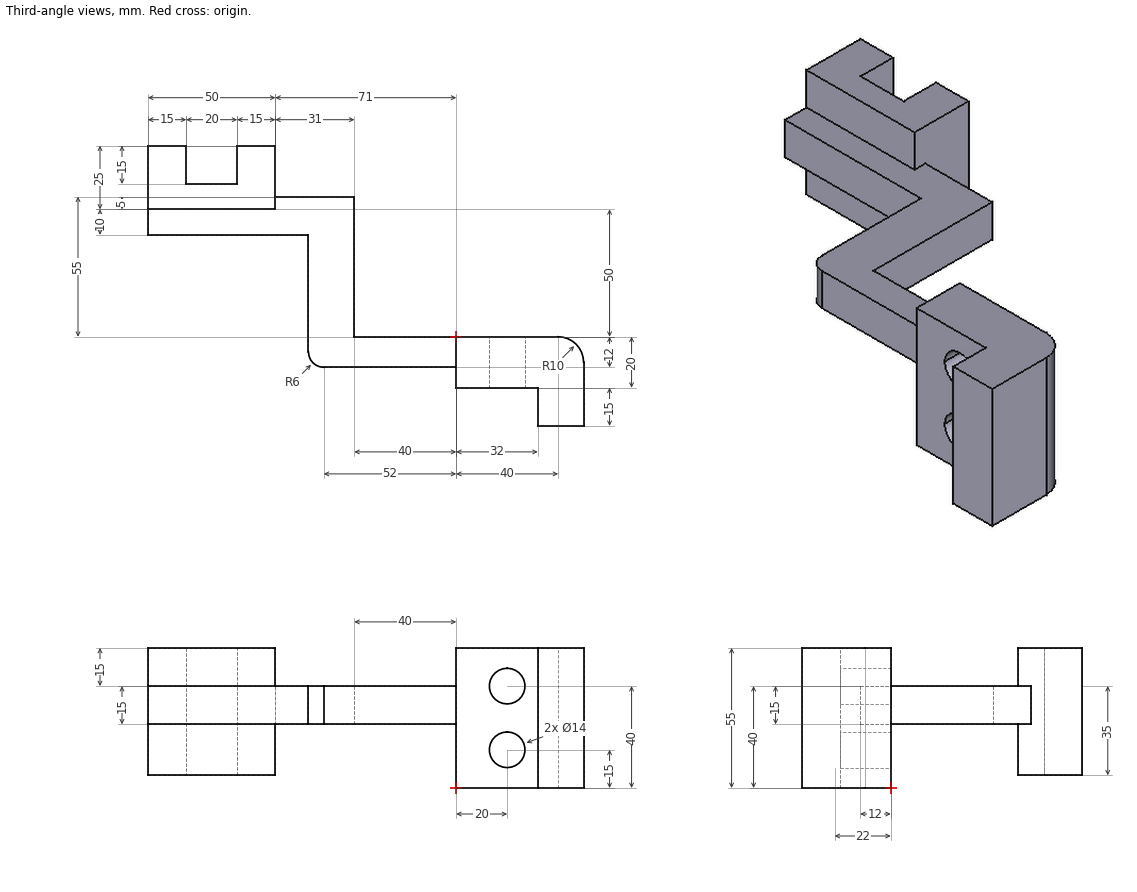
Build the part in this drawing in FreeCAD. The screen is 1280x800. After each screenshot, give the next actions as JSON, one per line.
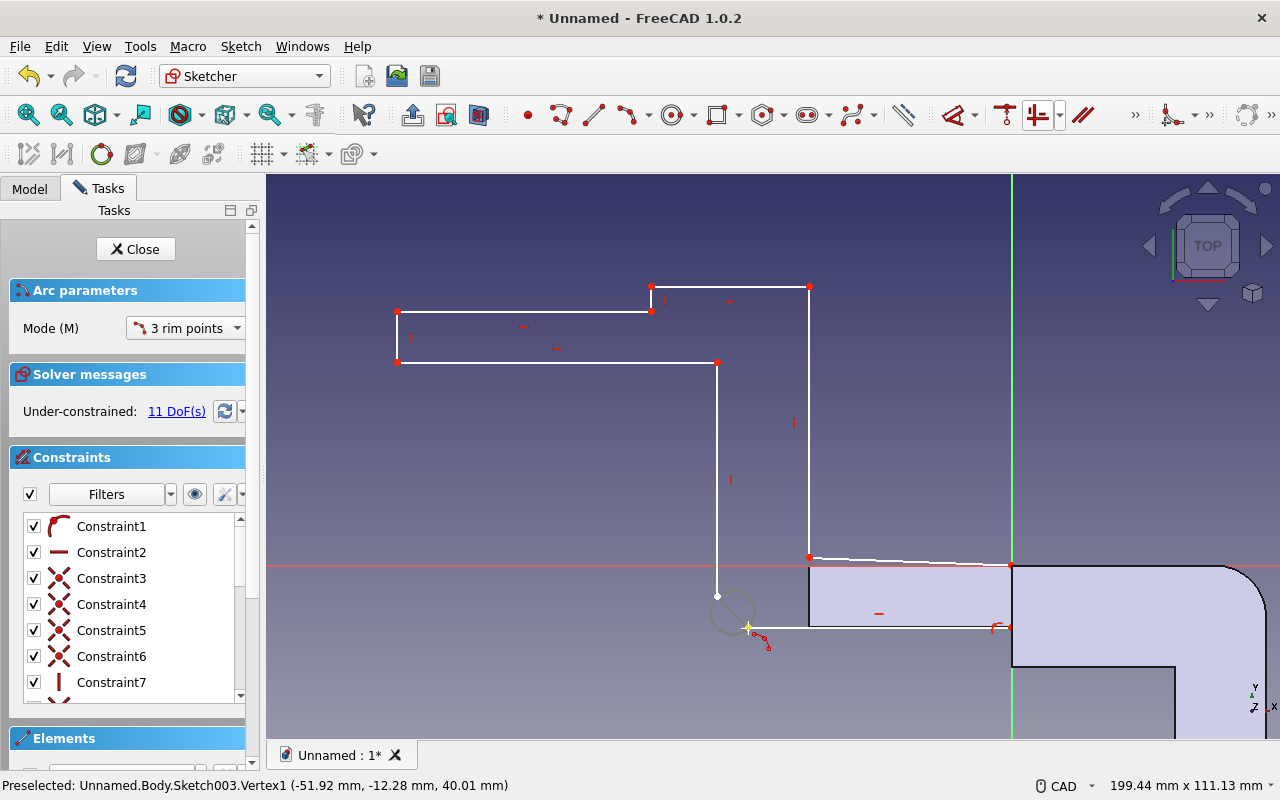
{"action": "scroll", "coordinate": [726, 618], "scroll_direction": "up", "scroll_amount": 3}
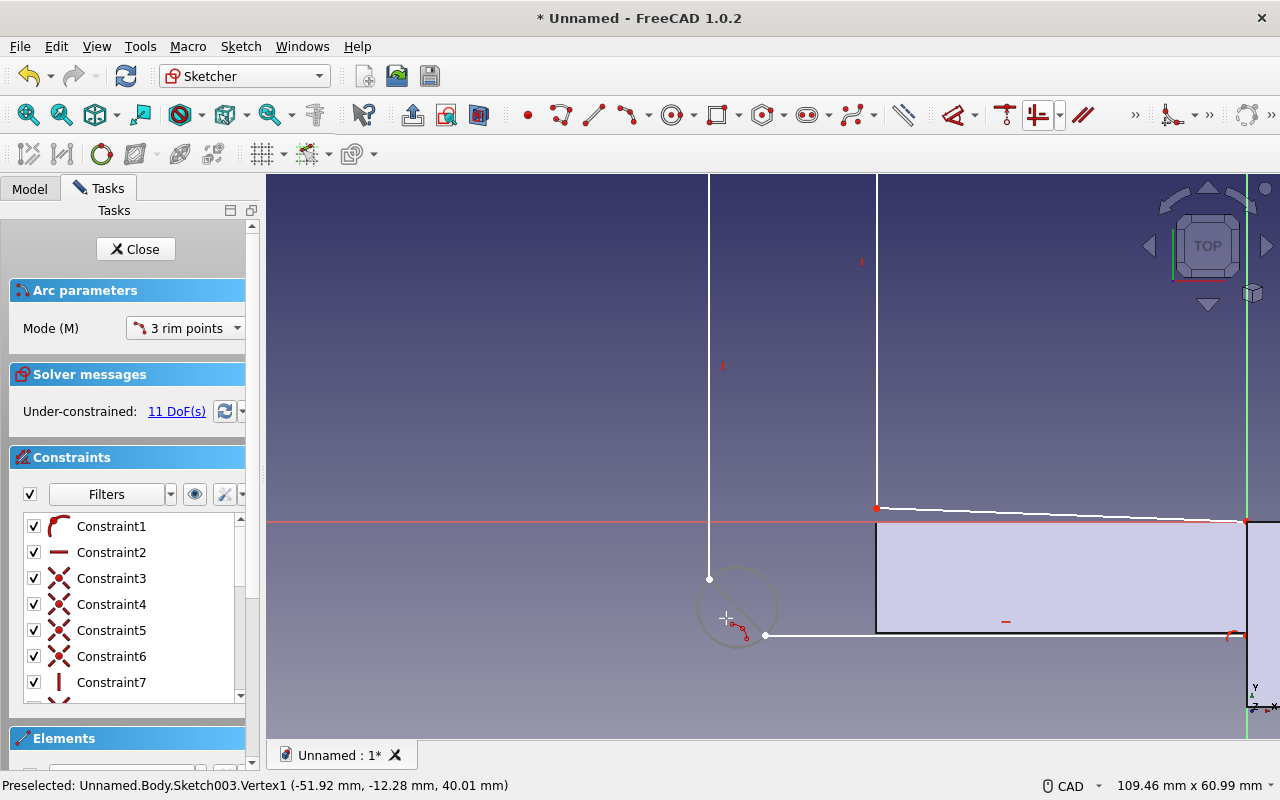
{"action": "left_click", "coordinate": [726, 617]}
{"action": "key", "text": "Escape"}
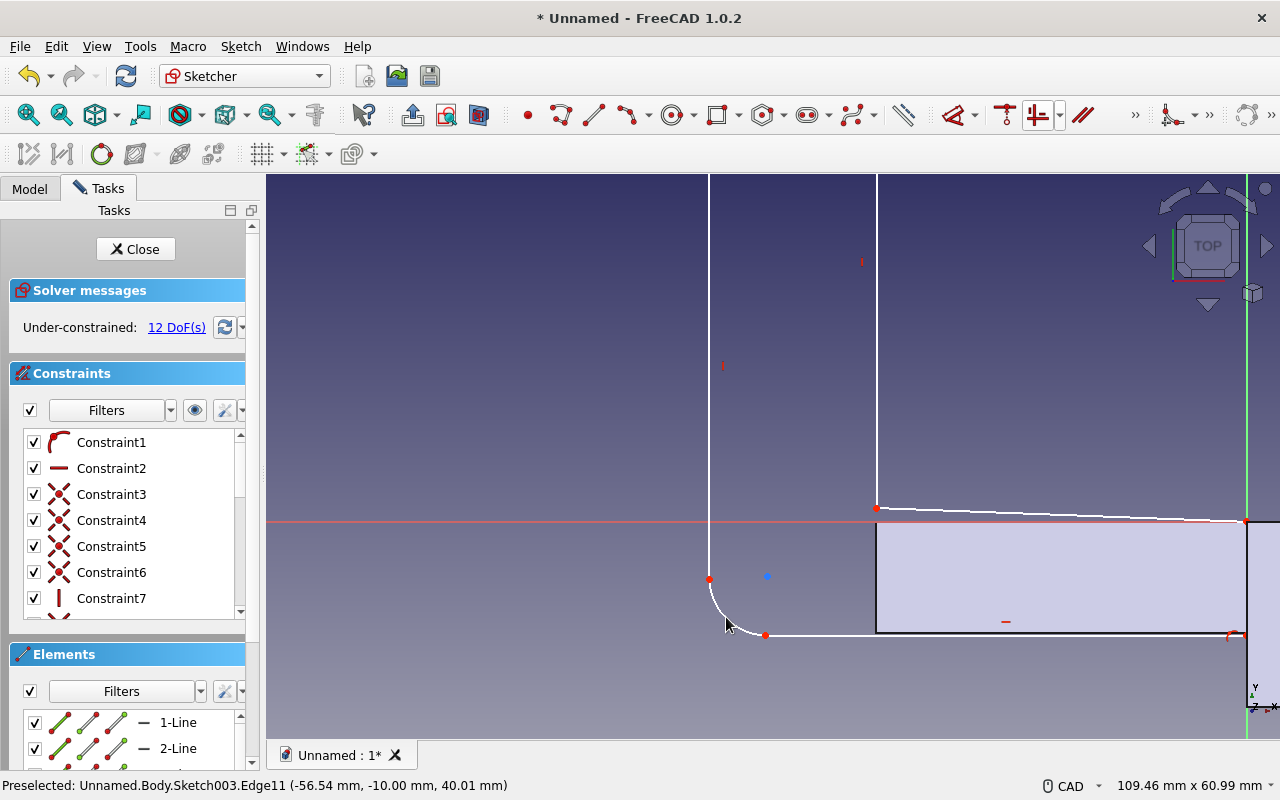
{"action": "left_click", "coordinate": [910, 636]}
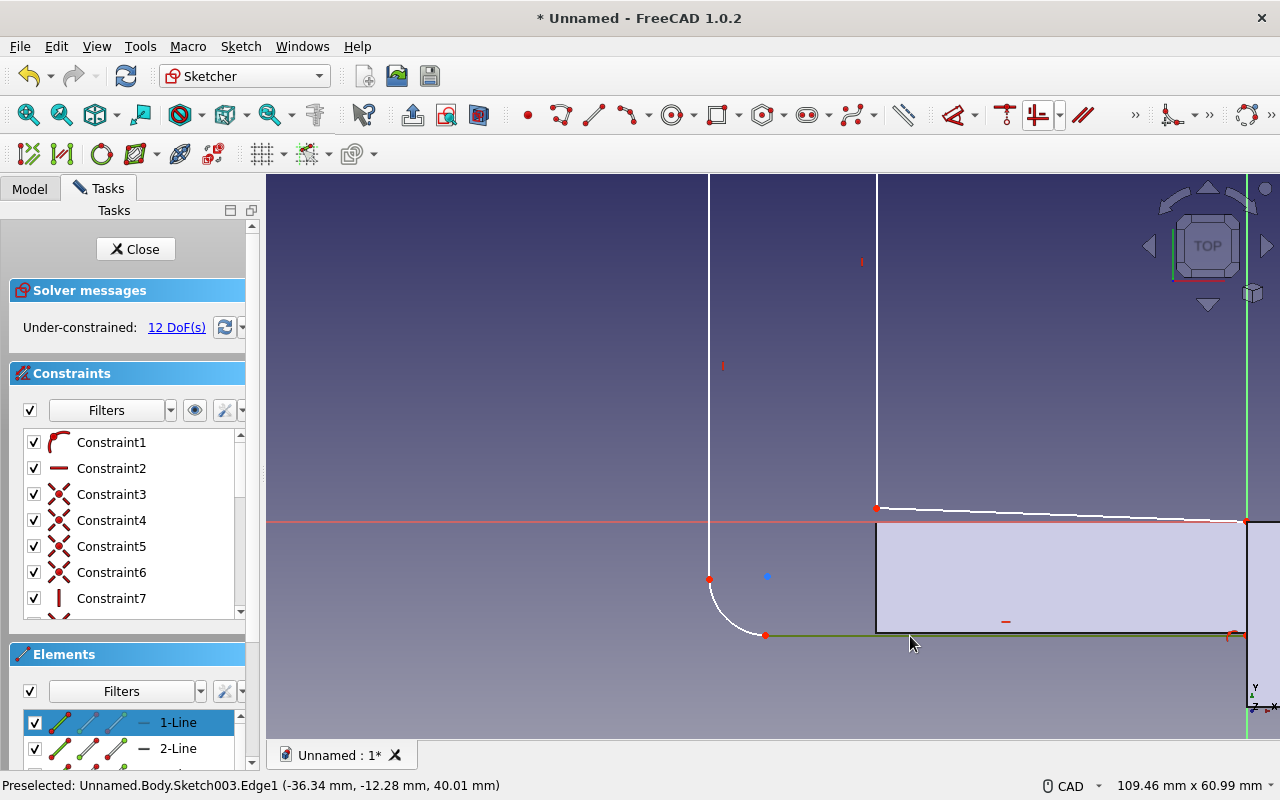
{"action": "left_click", "coordinate": [716, 604]}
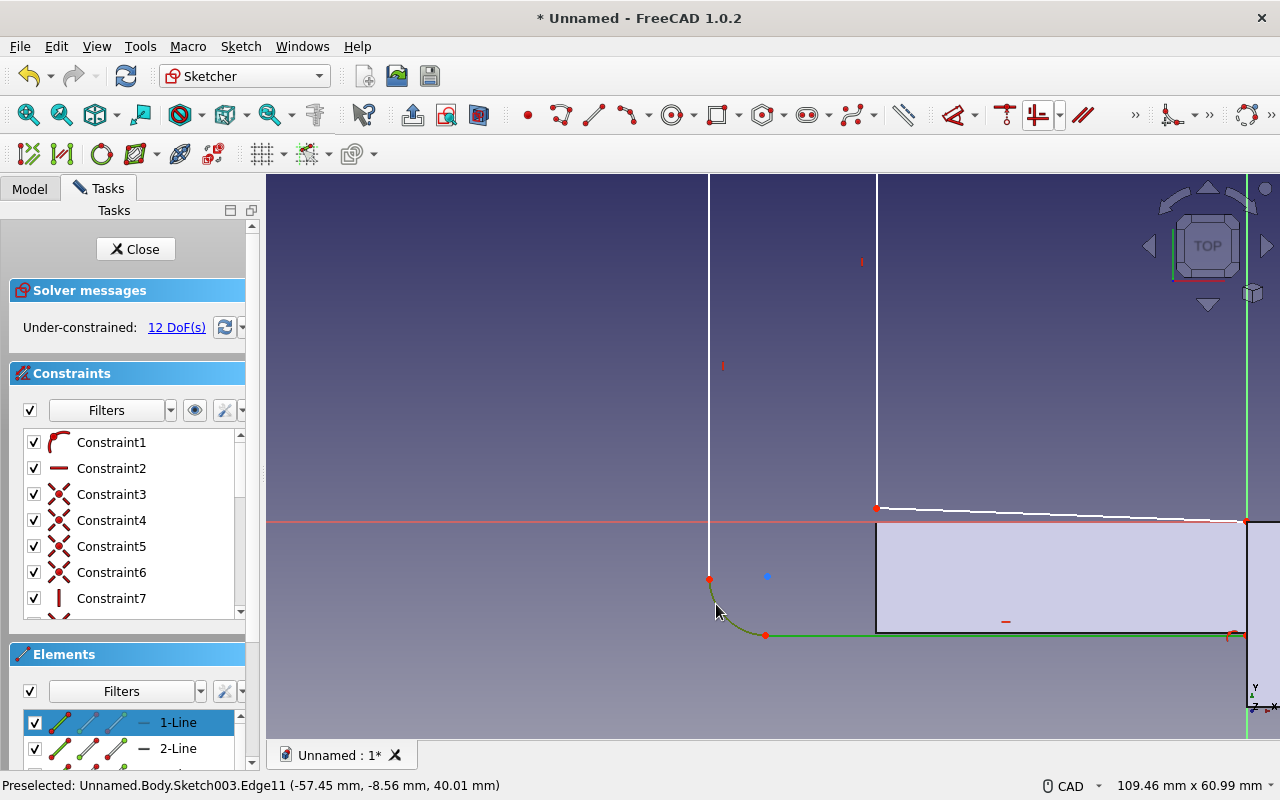
{"action": "key", "text": "t"}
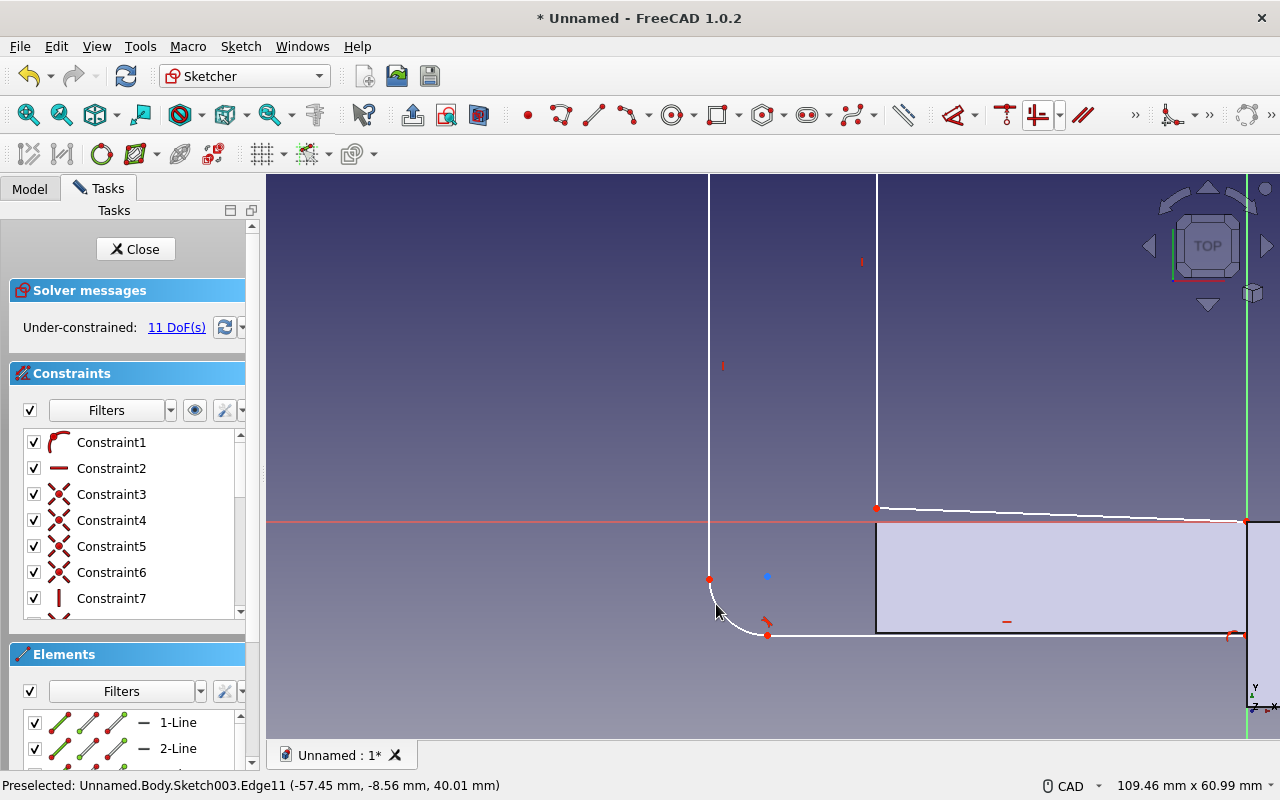
{"action": "left_click", "coordinate": [709, 281]}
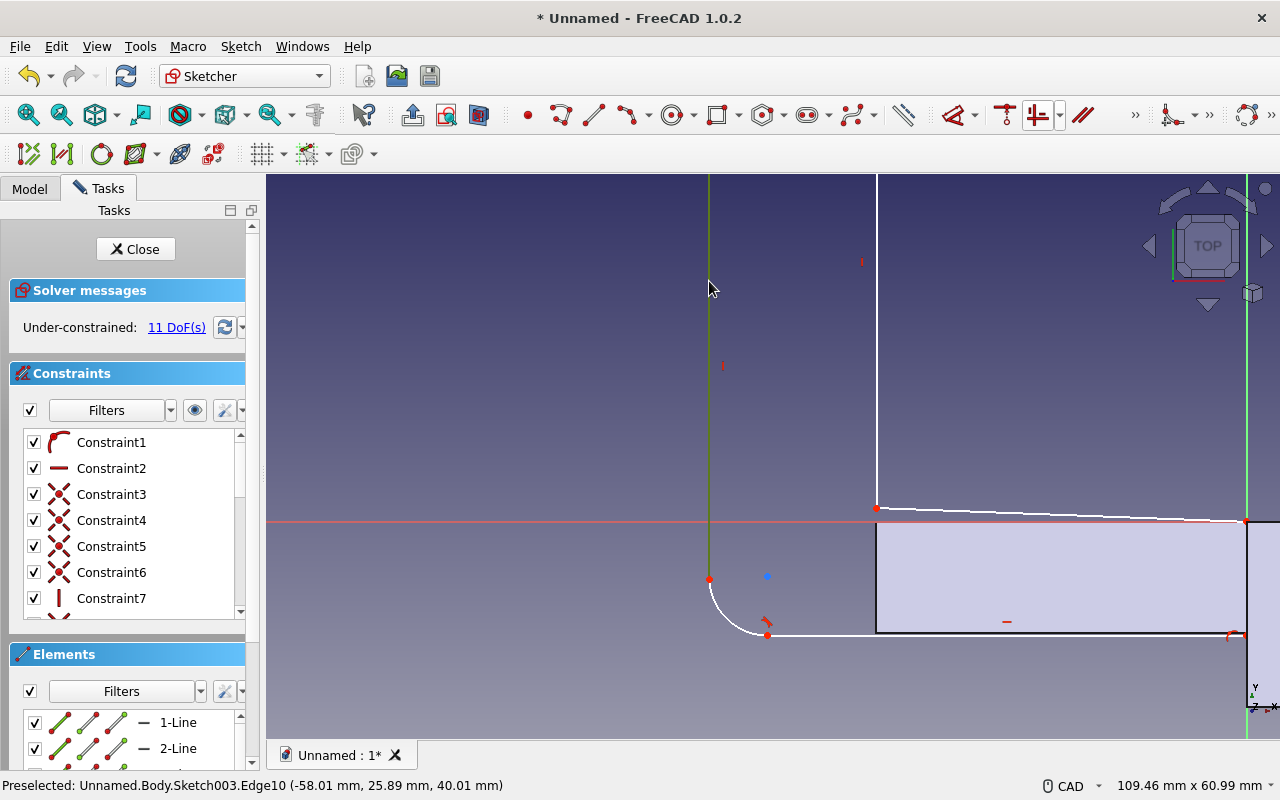
{"action": "left_click", "coordinate": [716, 605]}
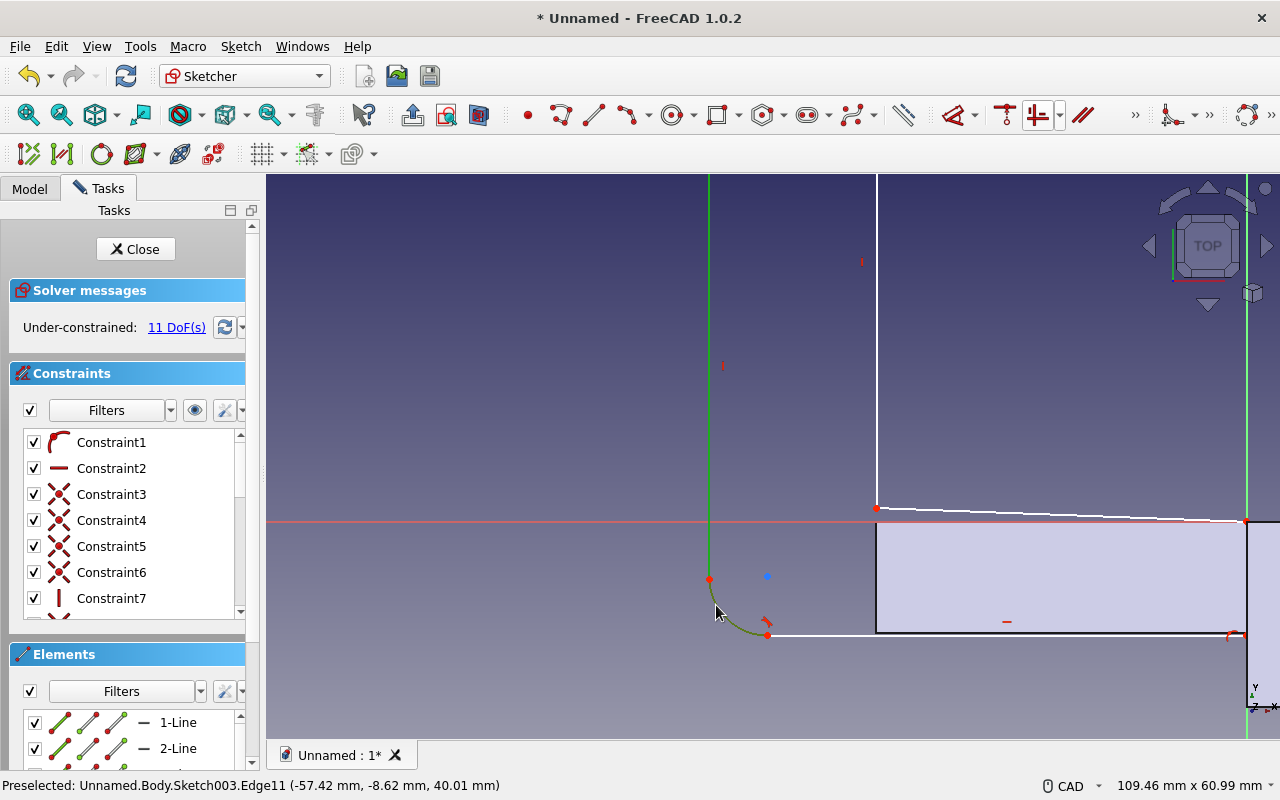
{"action": "key", "text": "t"}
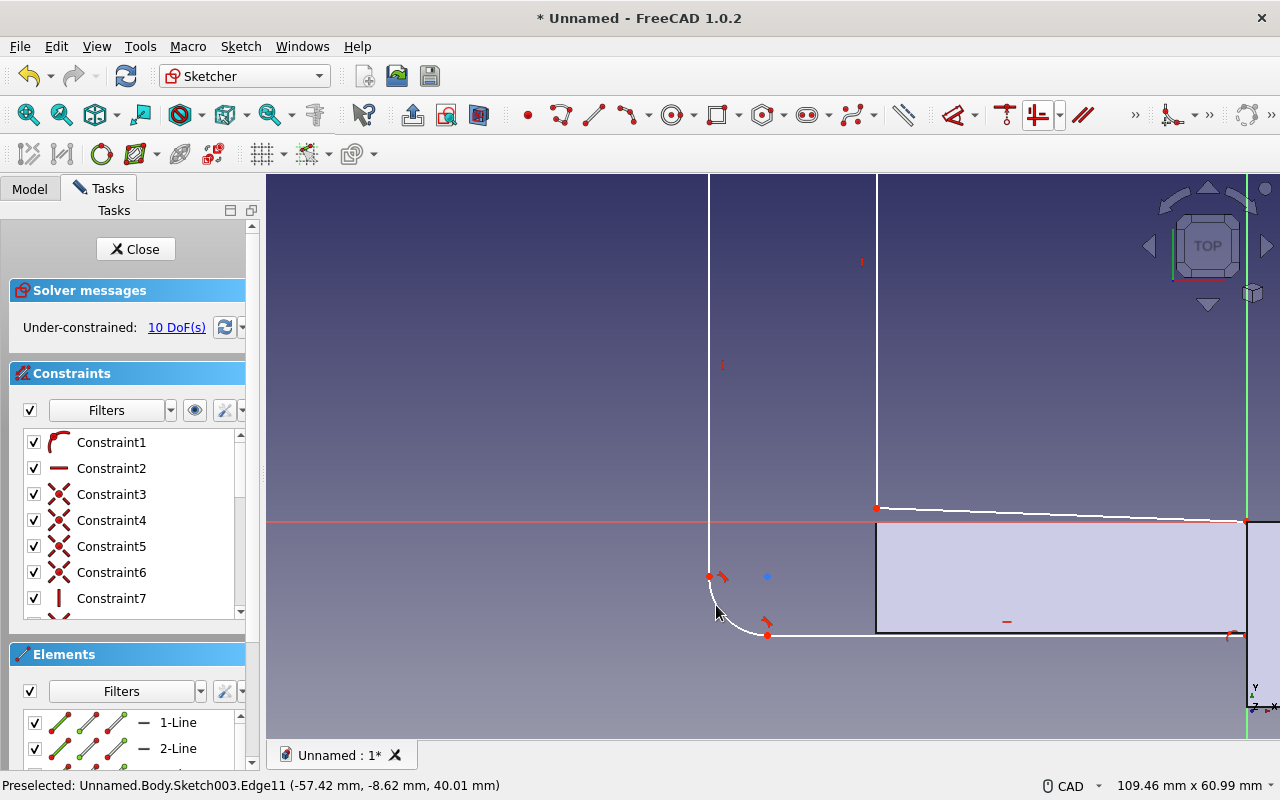
{"action": "scroll", "coordinate": [988, 512], "scroll_direction": "up", "scroll_amount": 2}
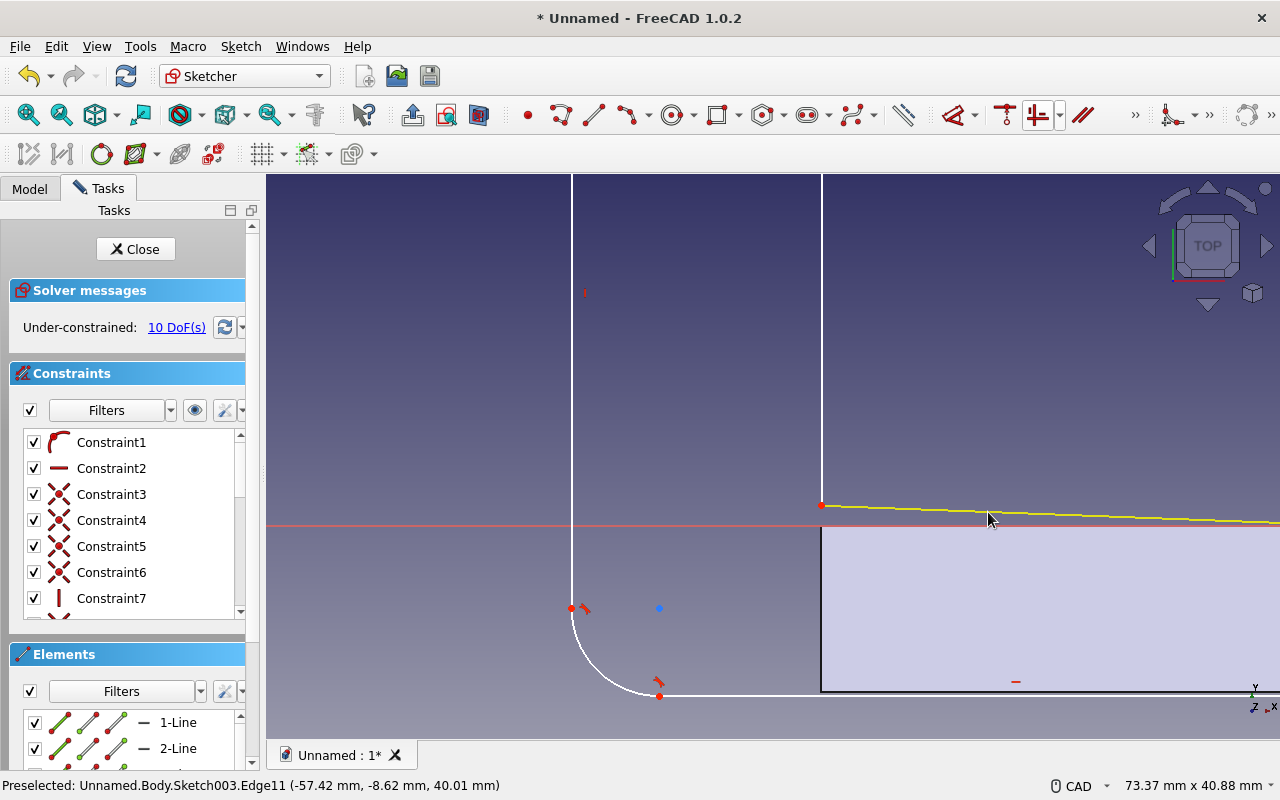
{"action": "left_click", "coordinate": [987, 512]}